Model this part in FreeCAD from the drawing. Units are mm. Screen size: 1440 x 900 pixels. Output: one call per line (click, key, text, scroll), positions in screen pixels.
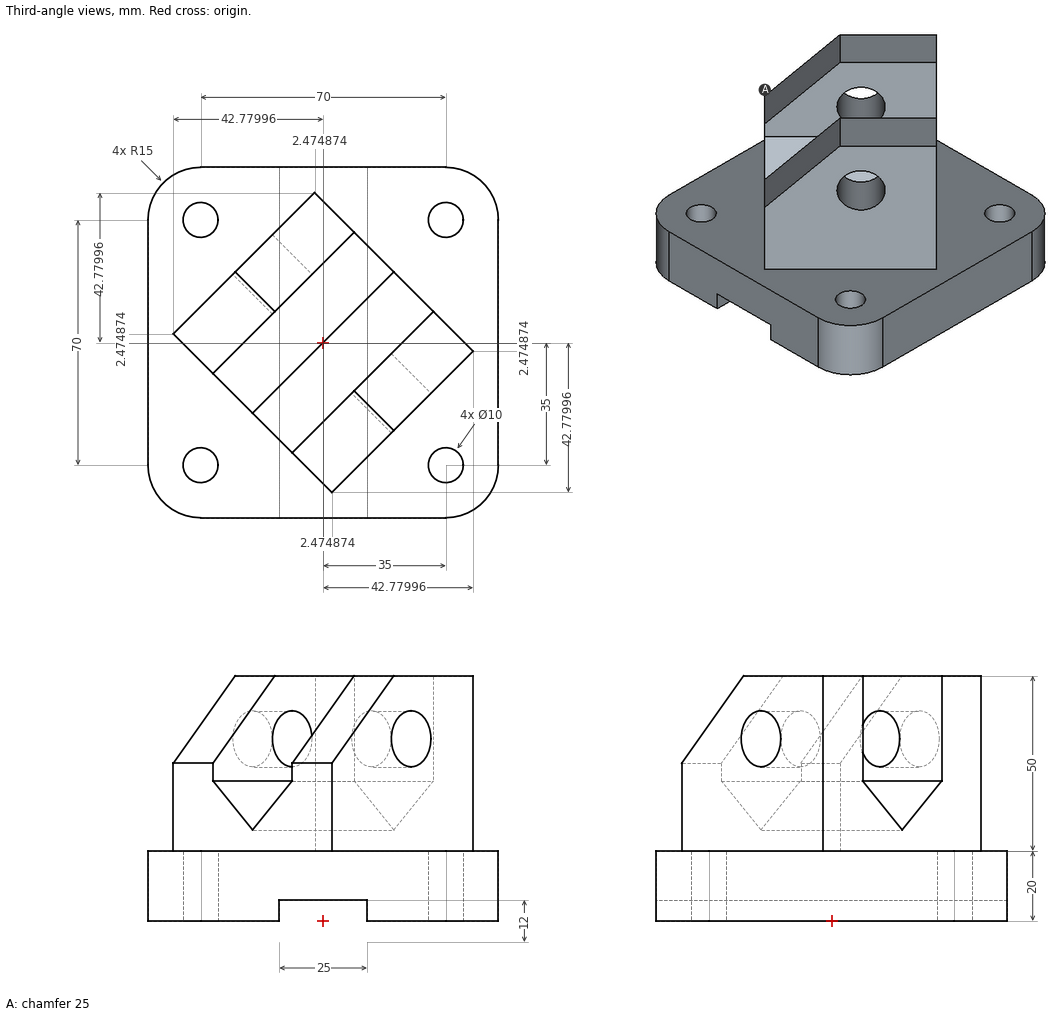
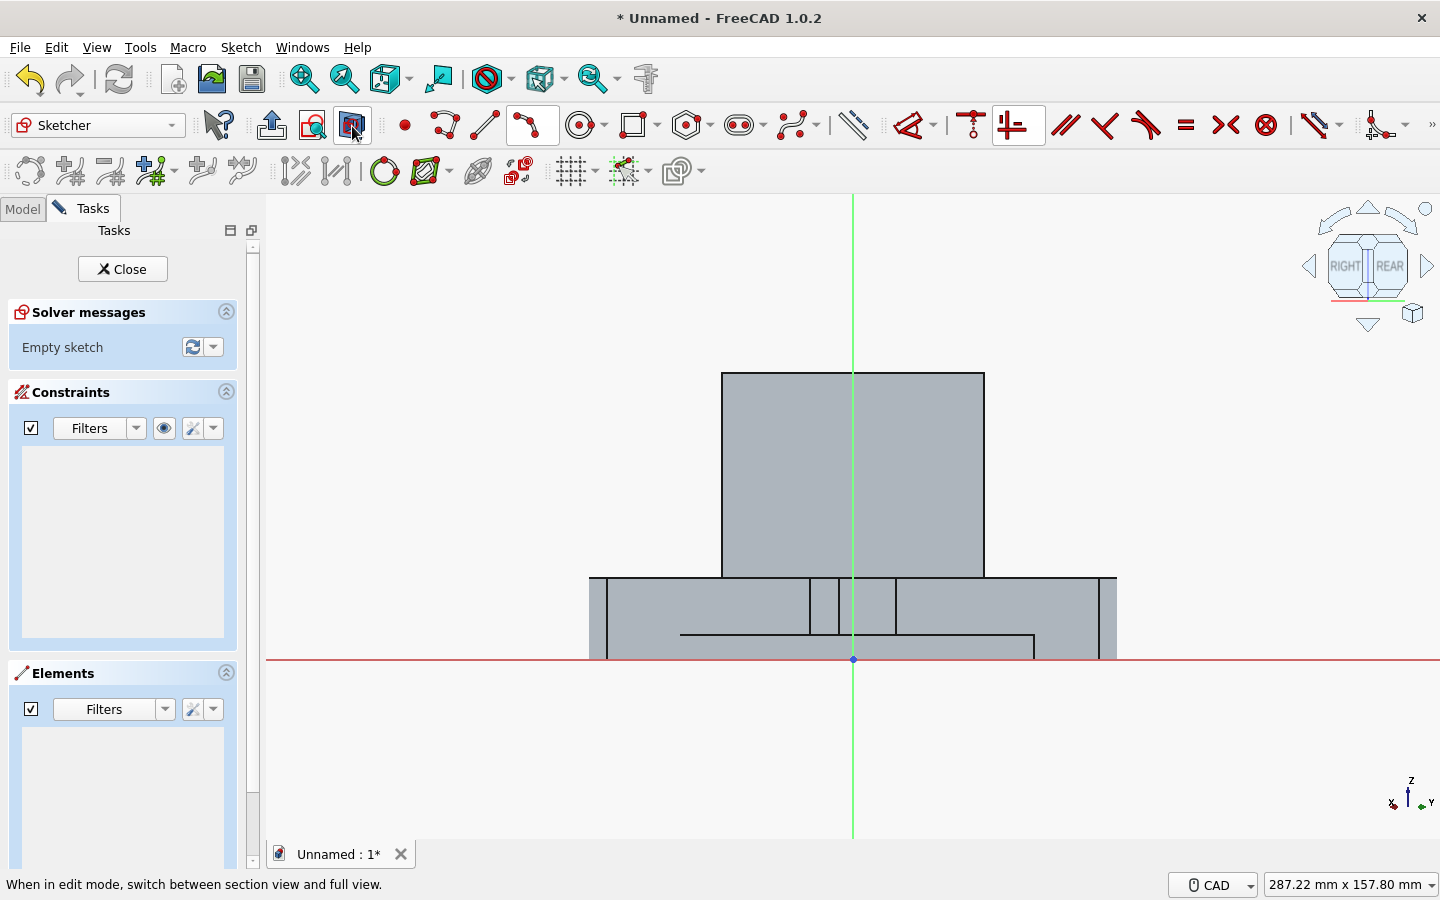
scroll(992, 516, up, 2)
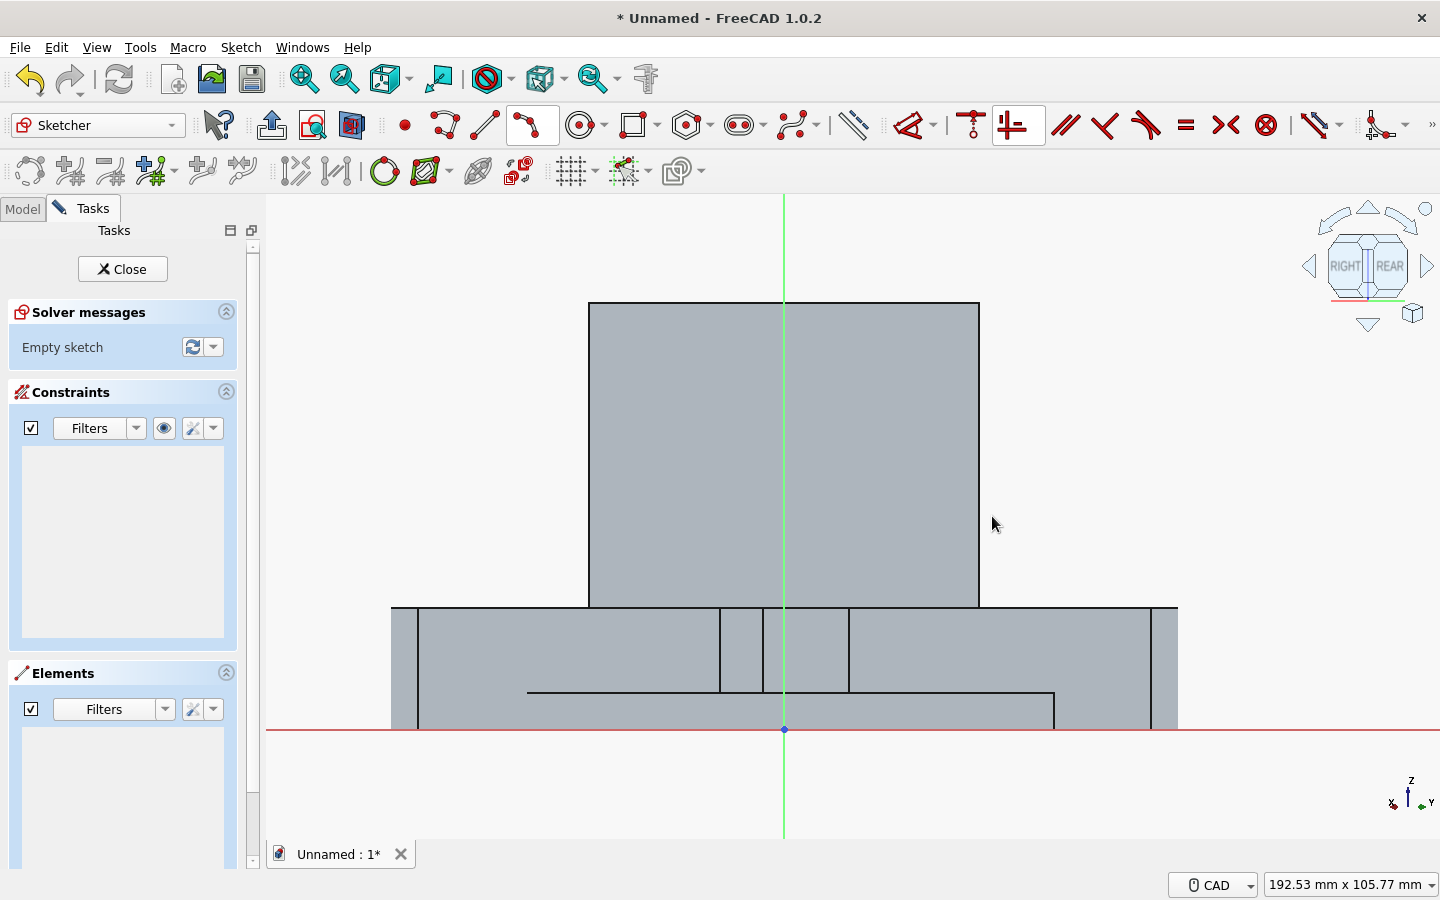
key(g)
key(m)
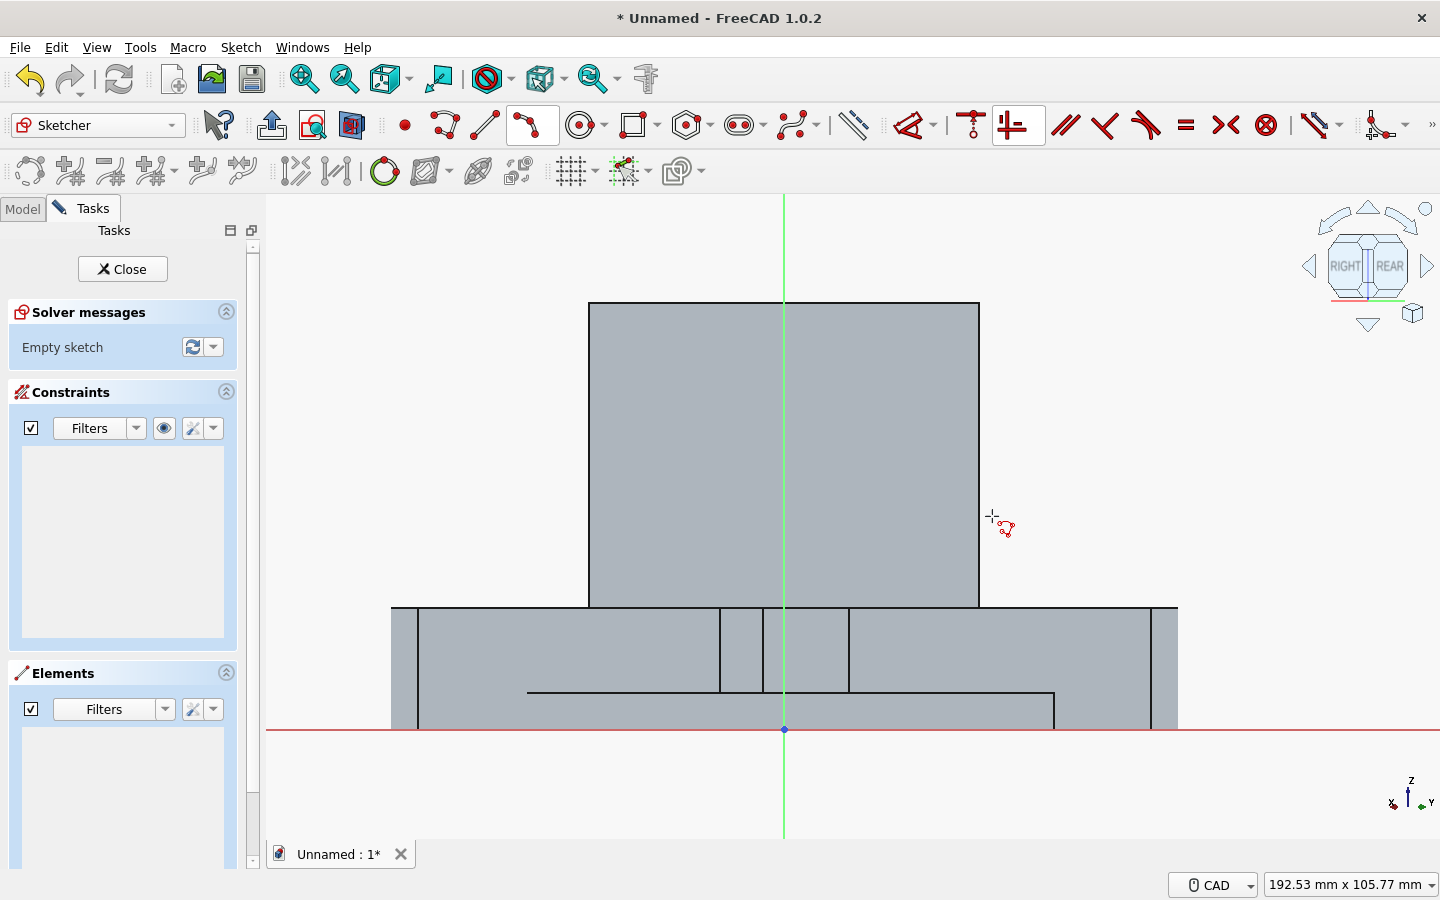
click(784, 571)
click(882, 486)
click(882, 303)
click(687, 303)
click(687, 486)
click(784, 572)
key(Escape)
key(Escape)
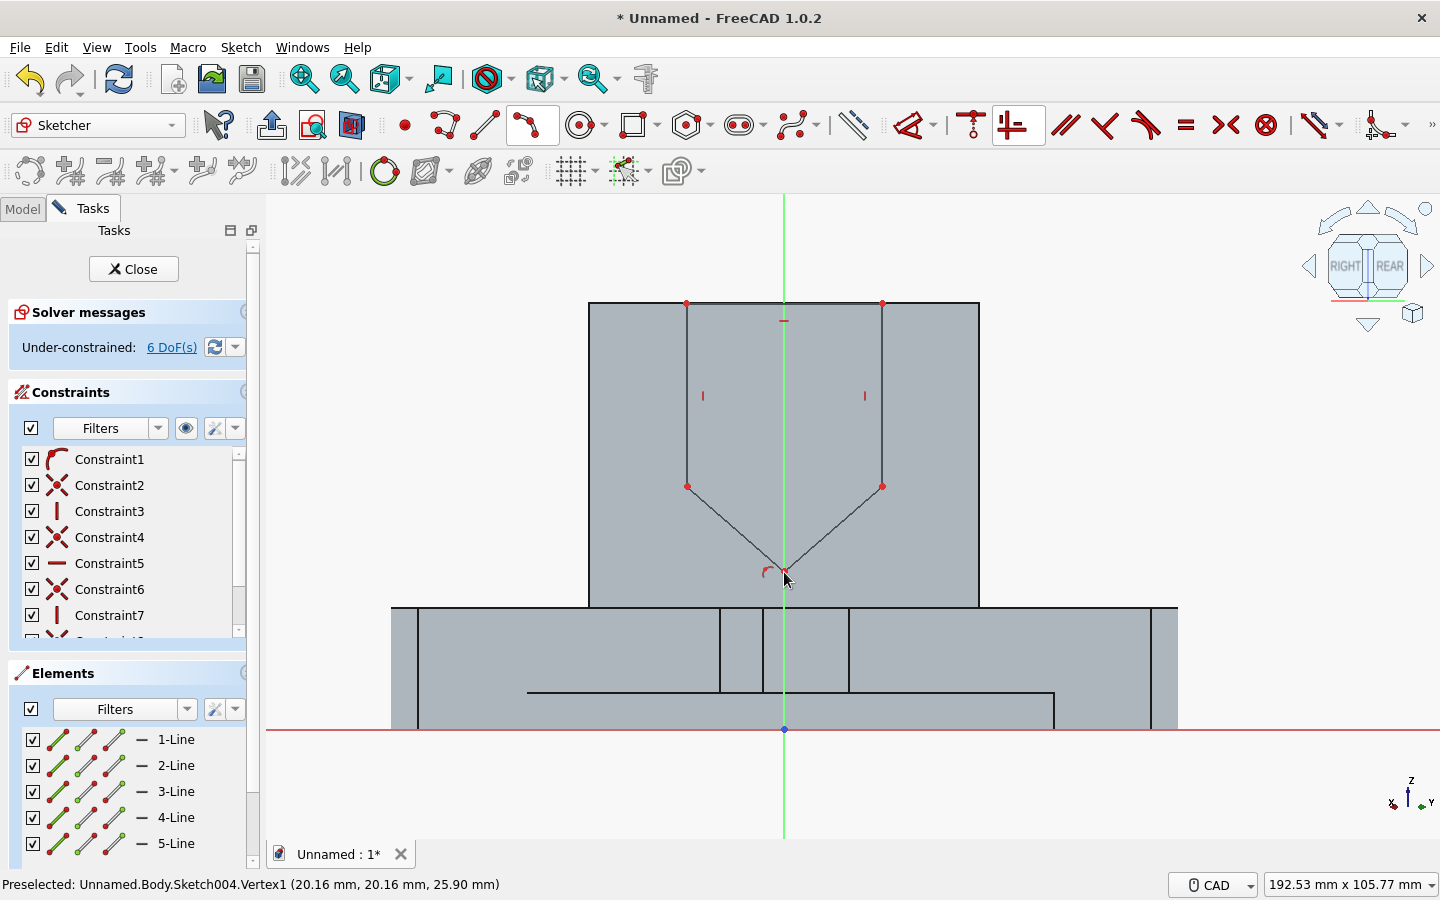
click(882, 487)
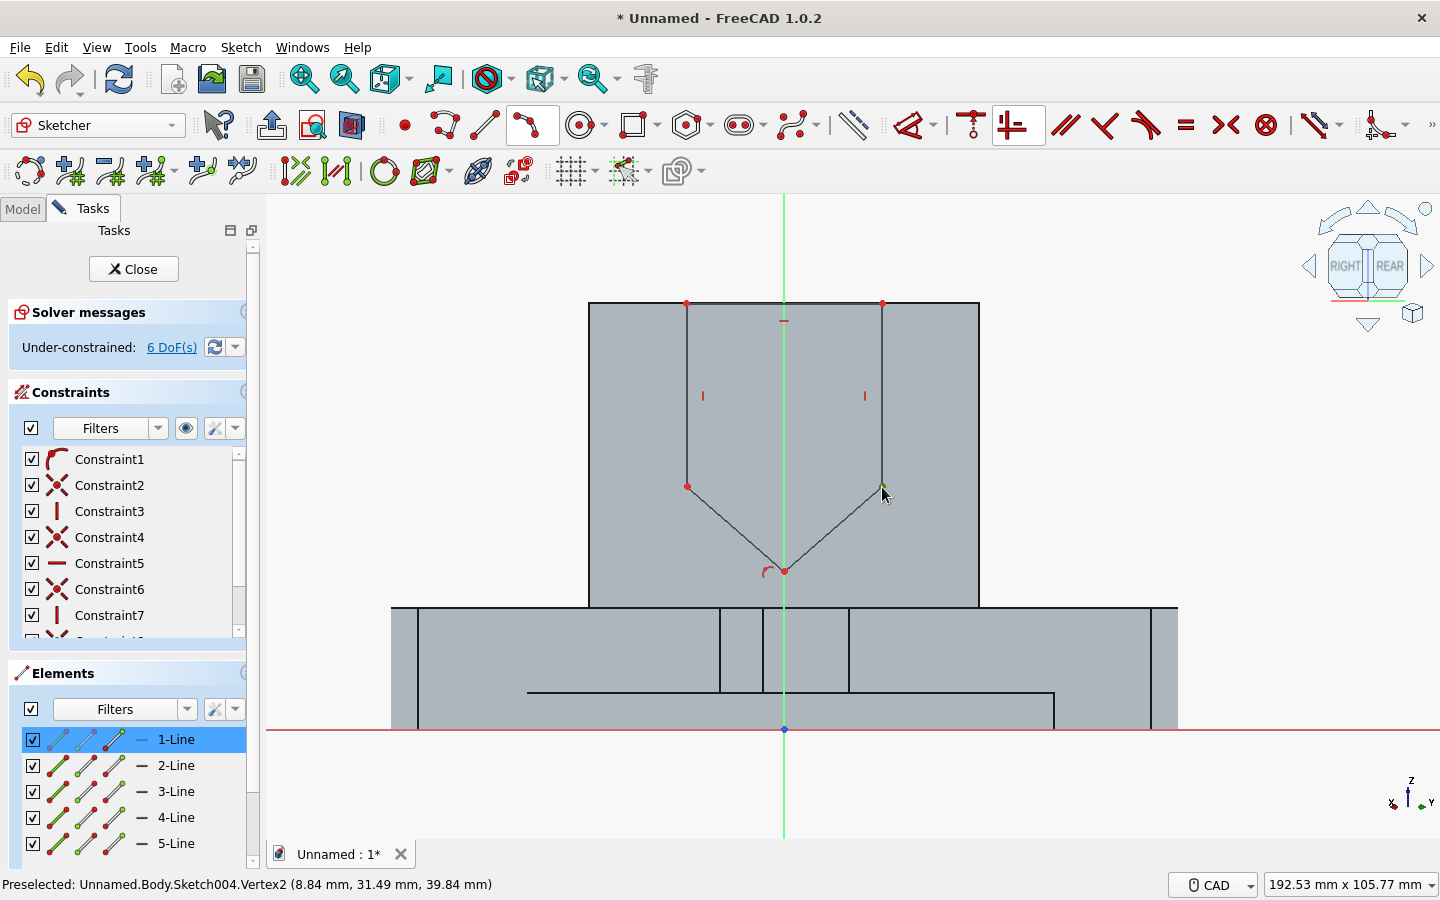
click(687, 487)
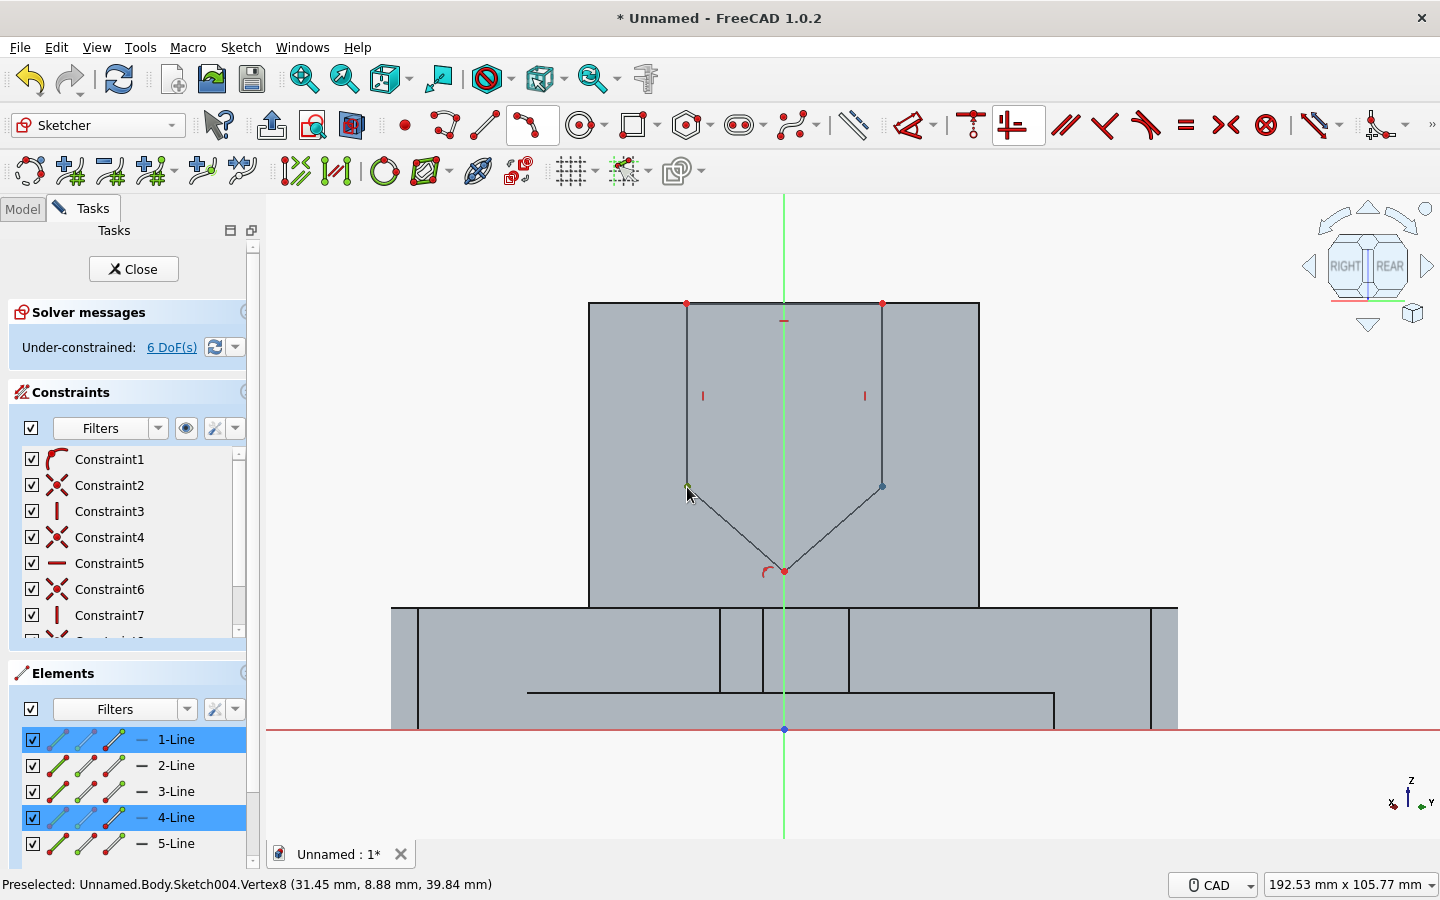
click(784, 769)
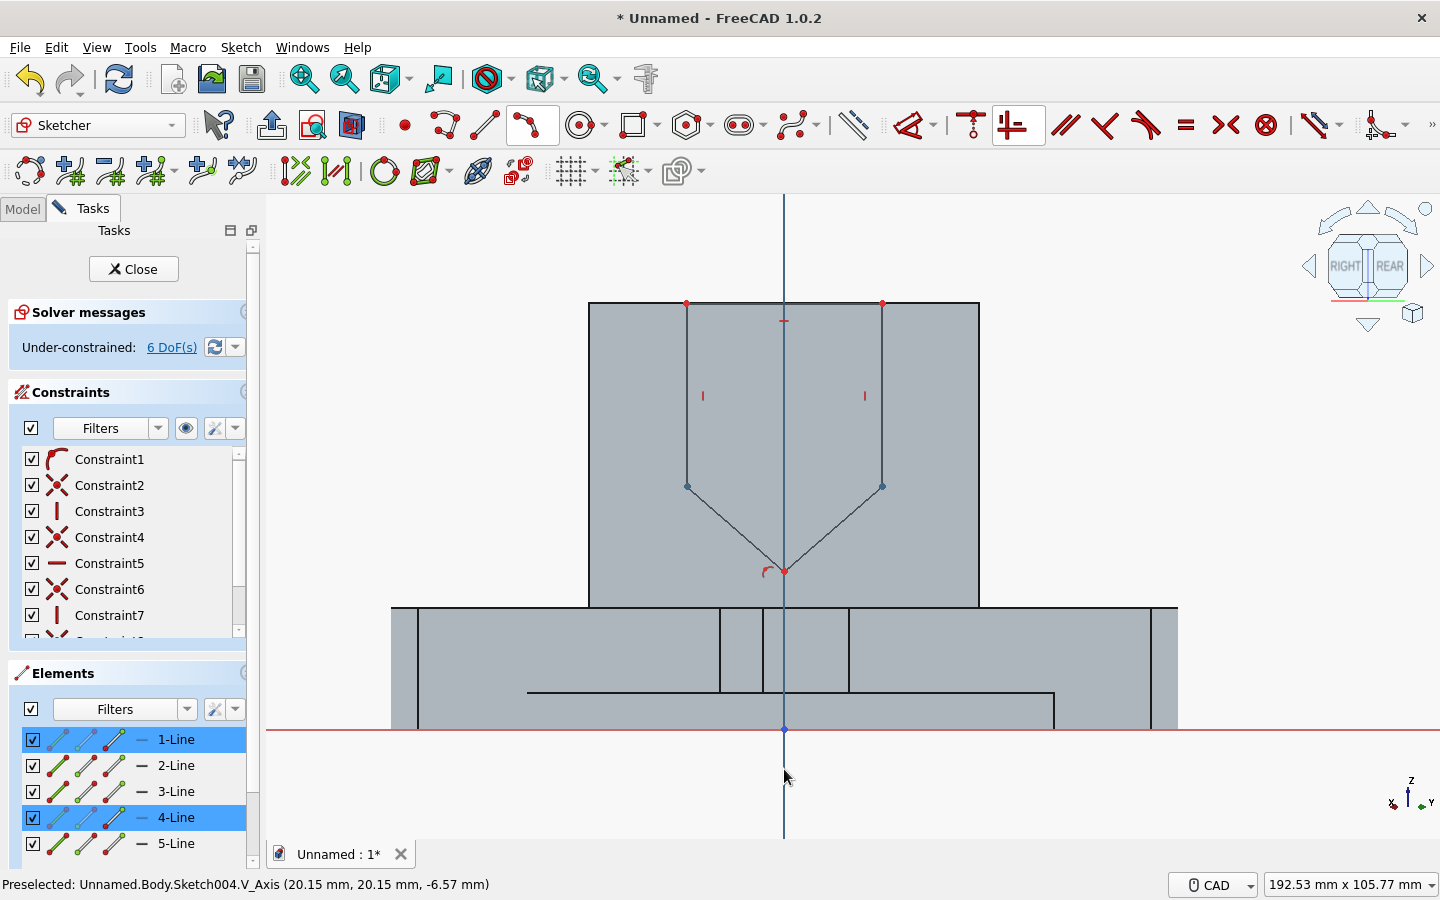
click(1226, 126)